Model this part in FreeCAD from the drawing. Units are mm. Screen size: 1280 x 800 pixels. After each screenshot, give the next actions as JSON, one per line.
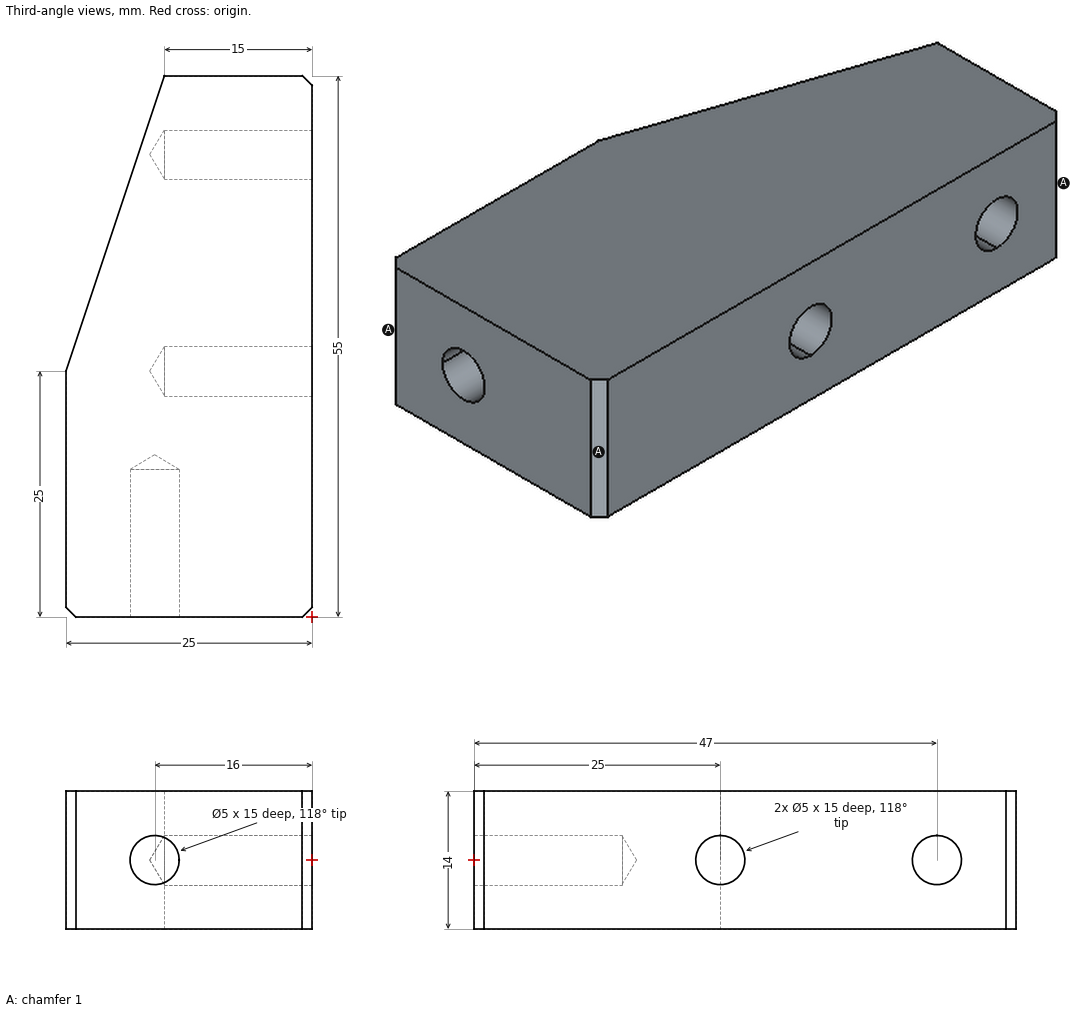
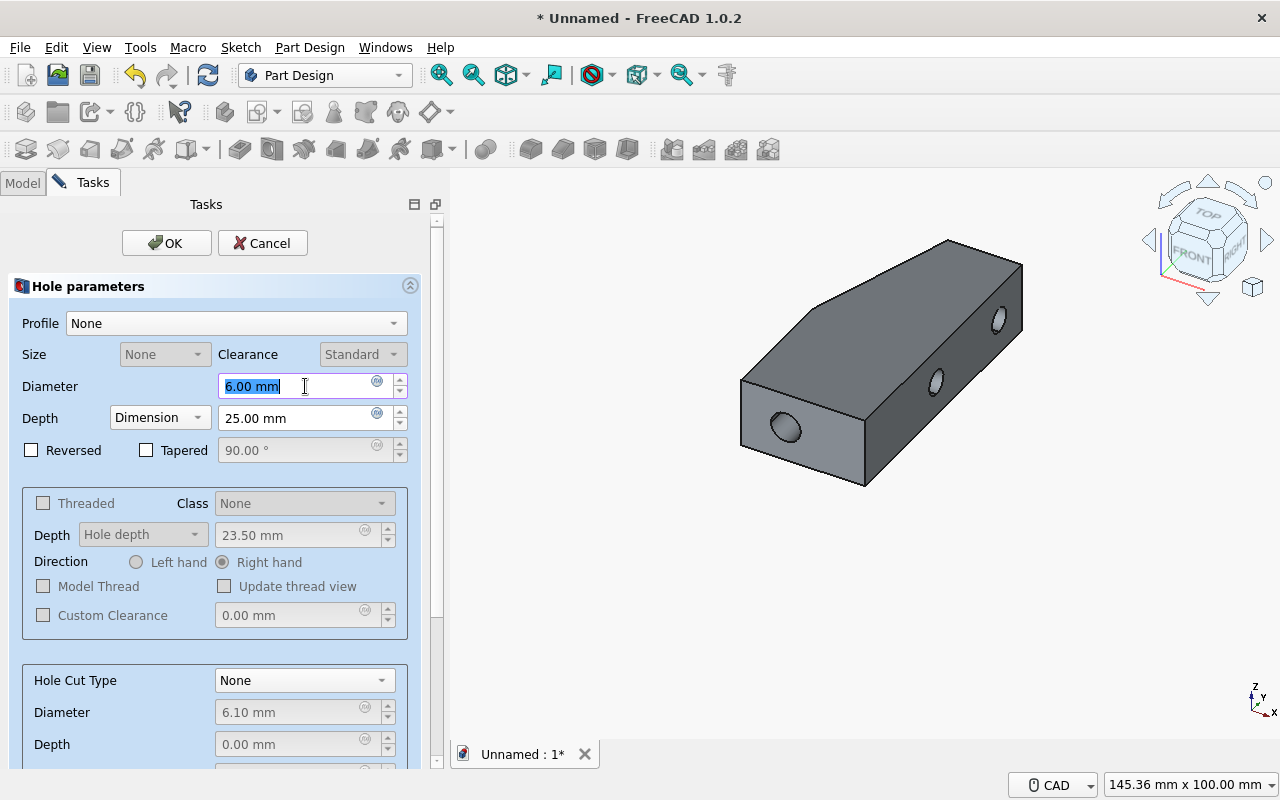
{"action": "type", "text": "5"}
{"action": "key", "text": "Tab"}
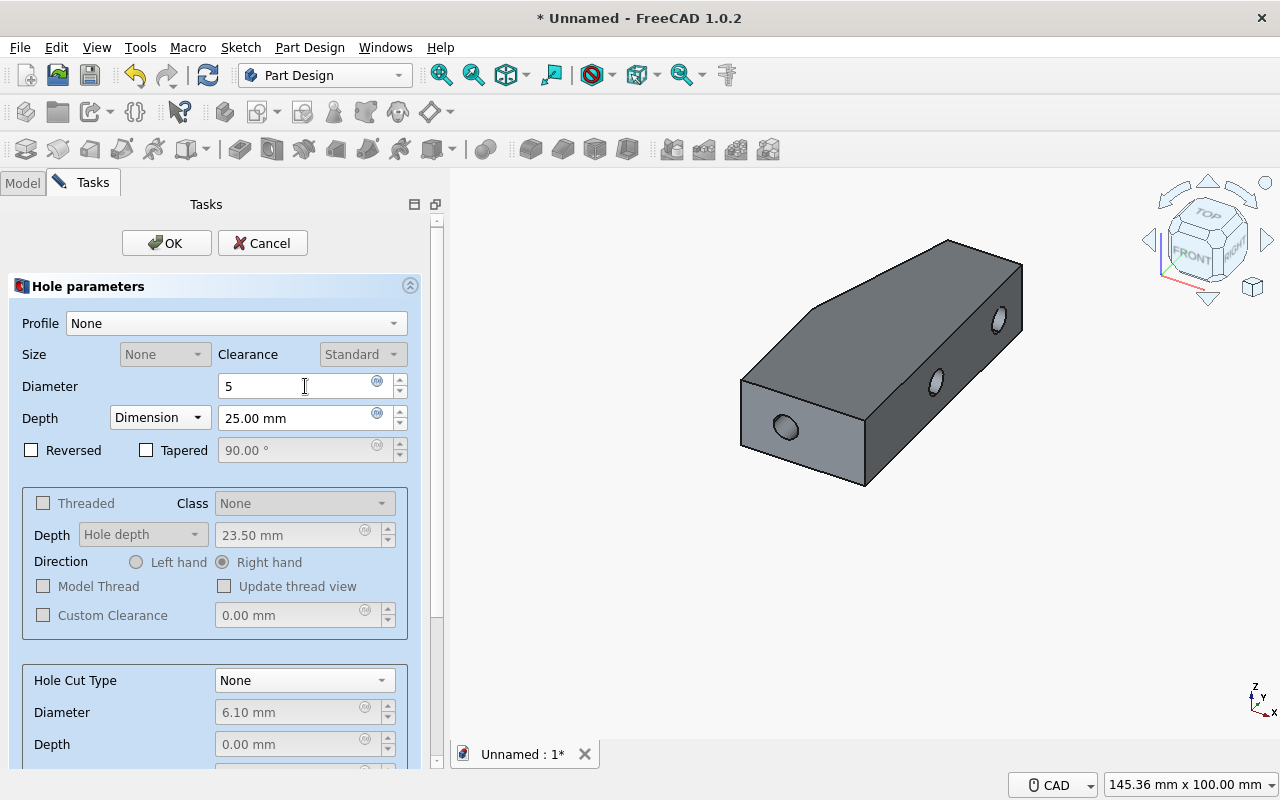
{"action": "triple_click", "coordinate": [305, 418]}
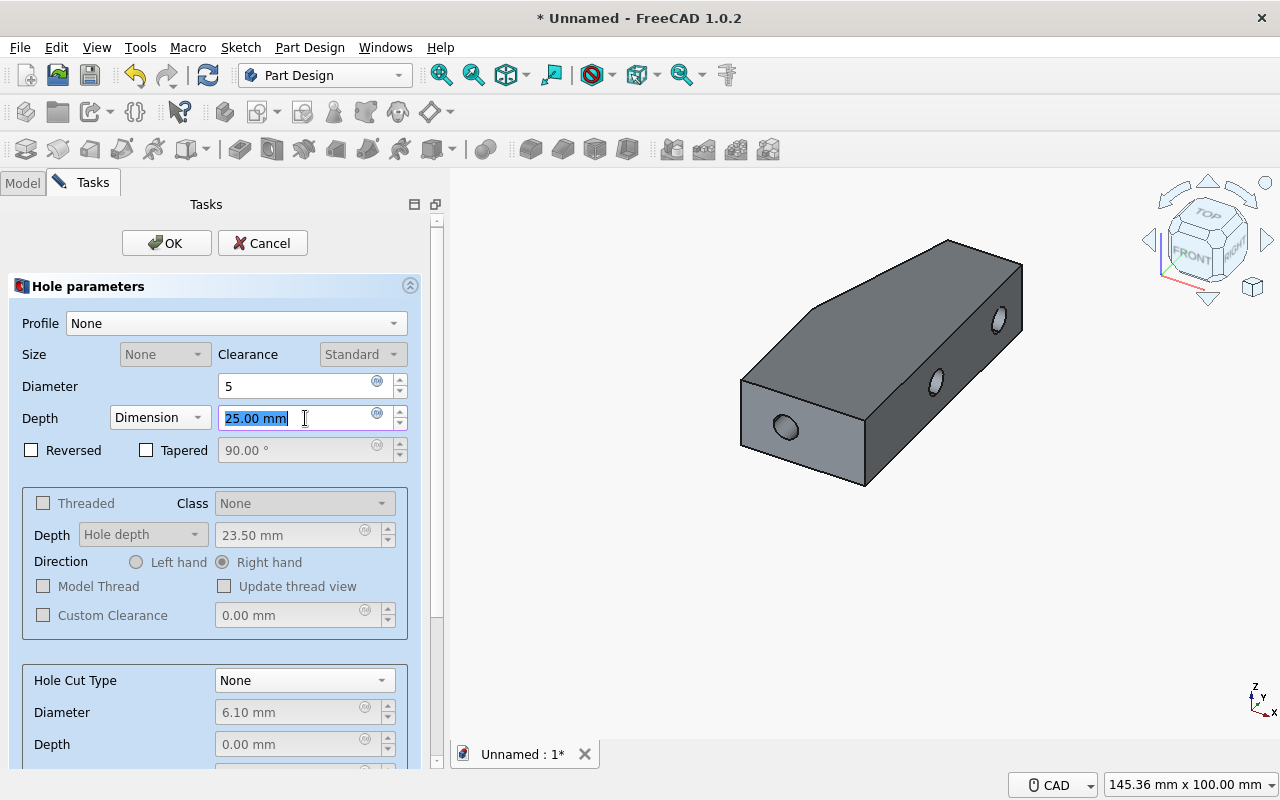
{"action": "type", "text": "15"}
{"action": "key", "text": "Tab"}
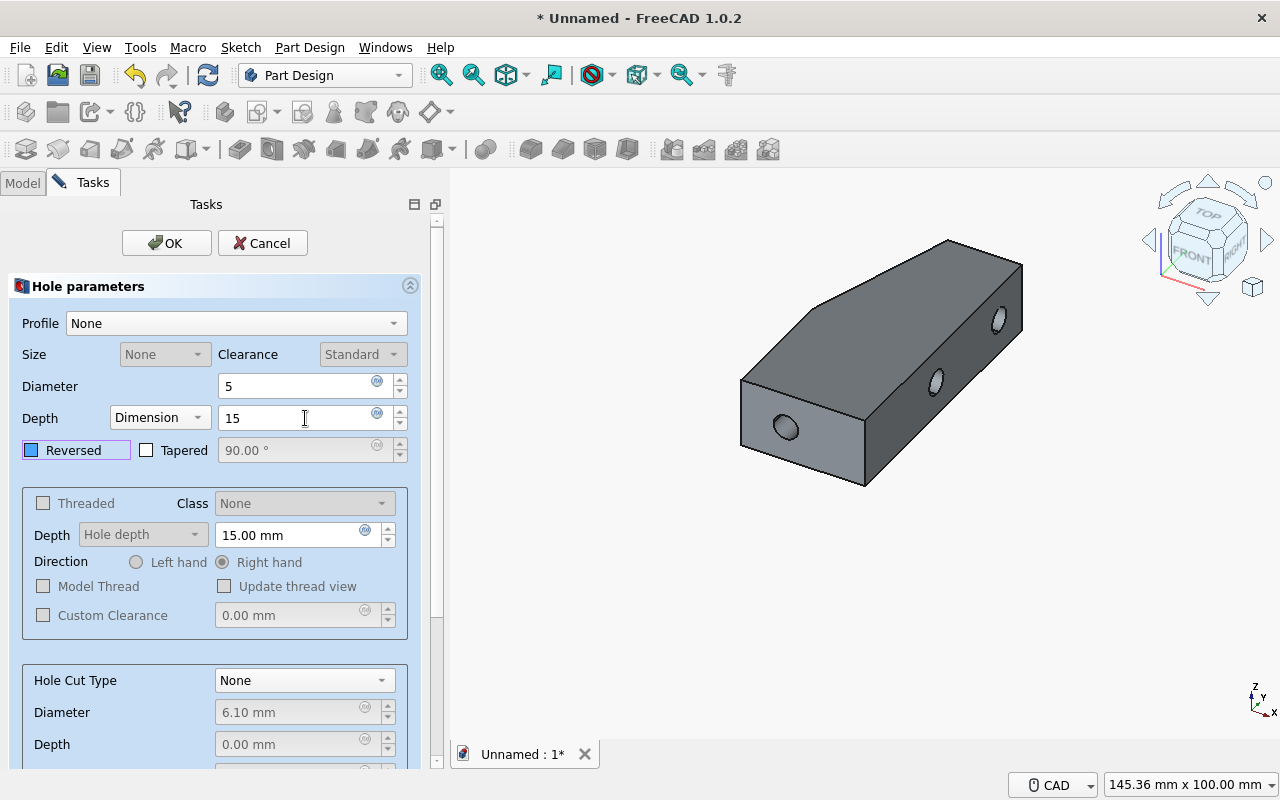
{"action": "left_click", "coordinate": [167, 243]}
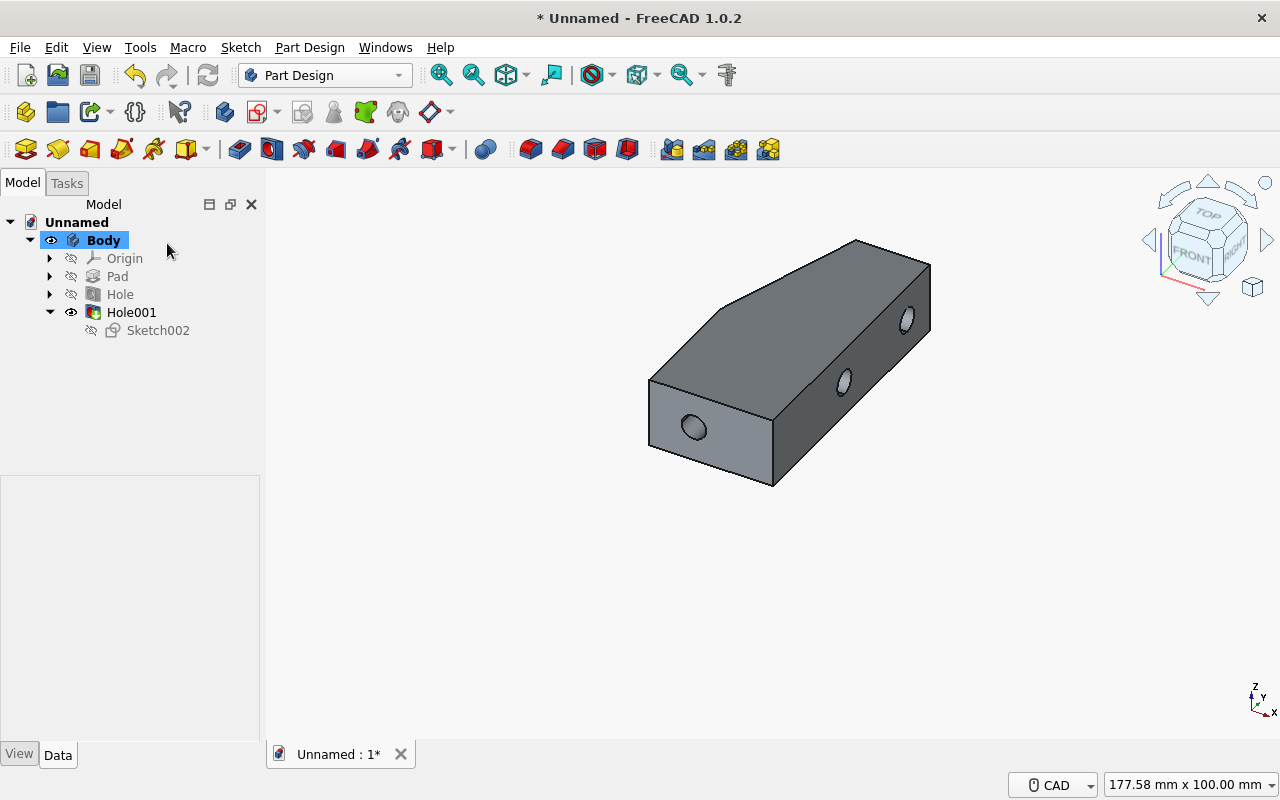
{"action": "left_click", "coordinate": [773, 452]}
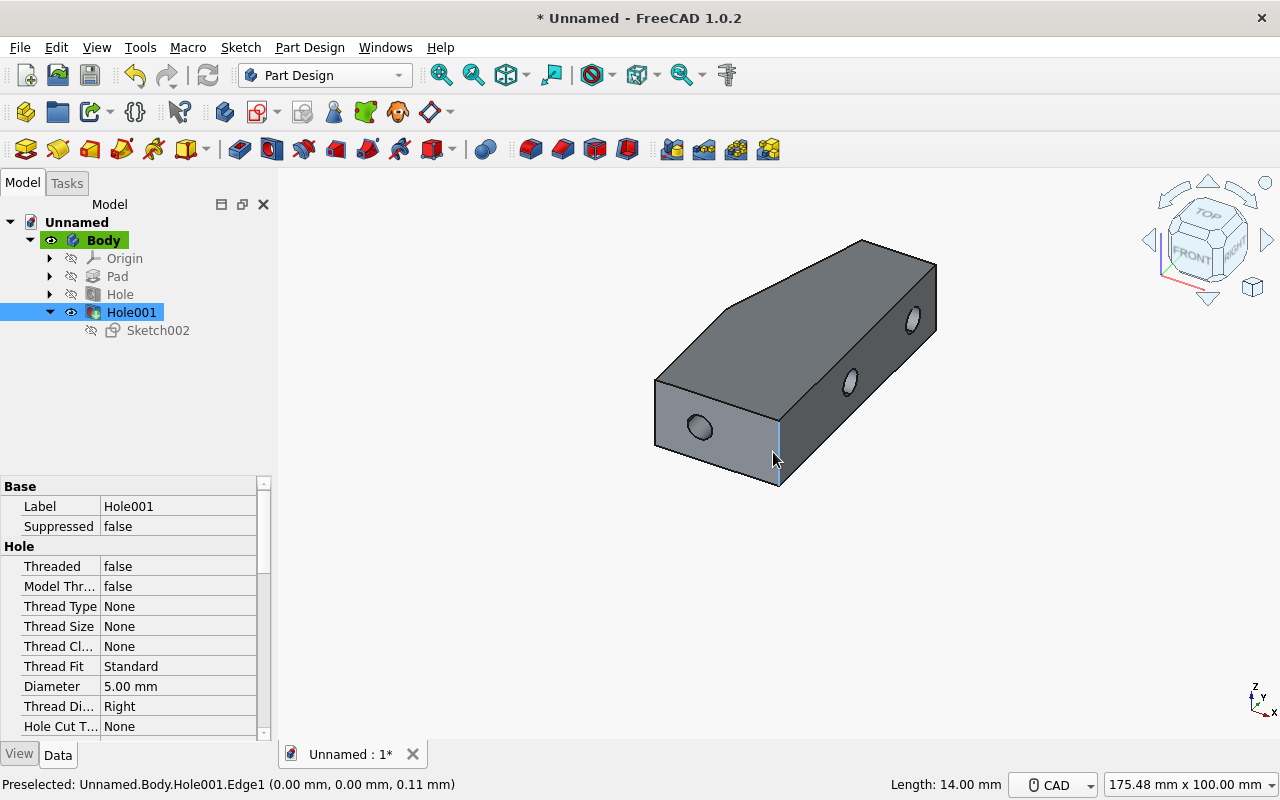
{"action": "key", "text": "0"}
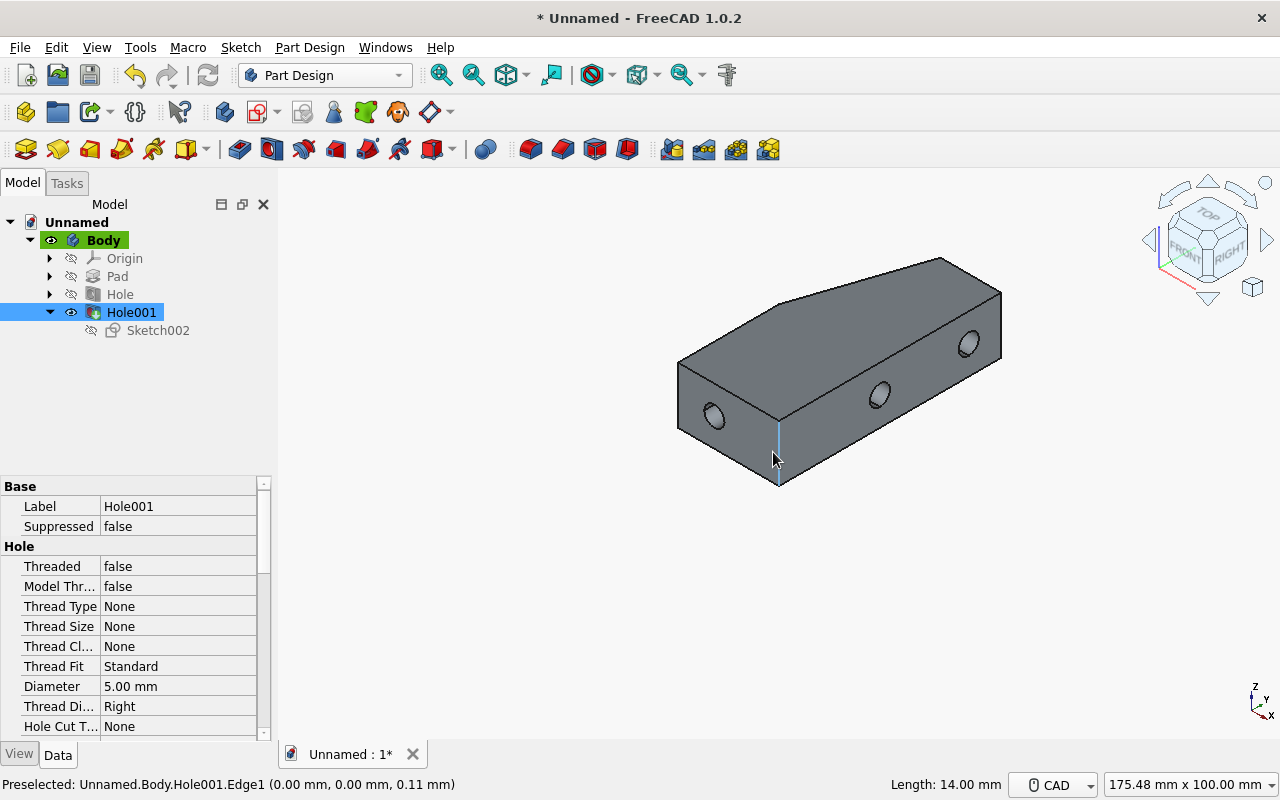
{"action": "key", "text": "v f"}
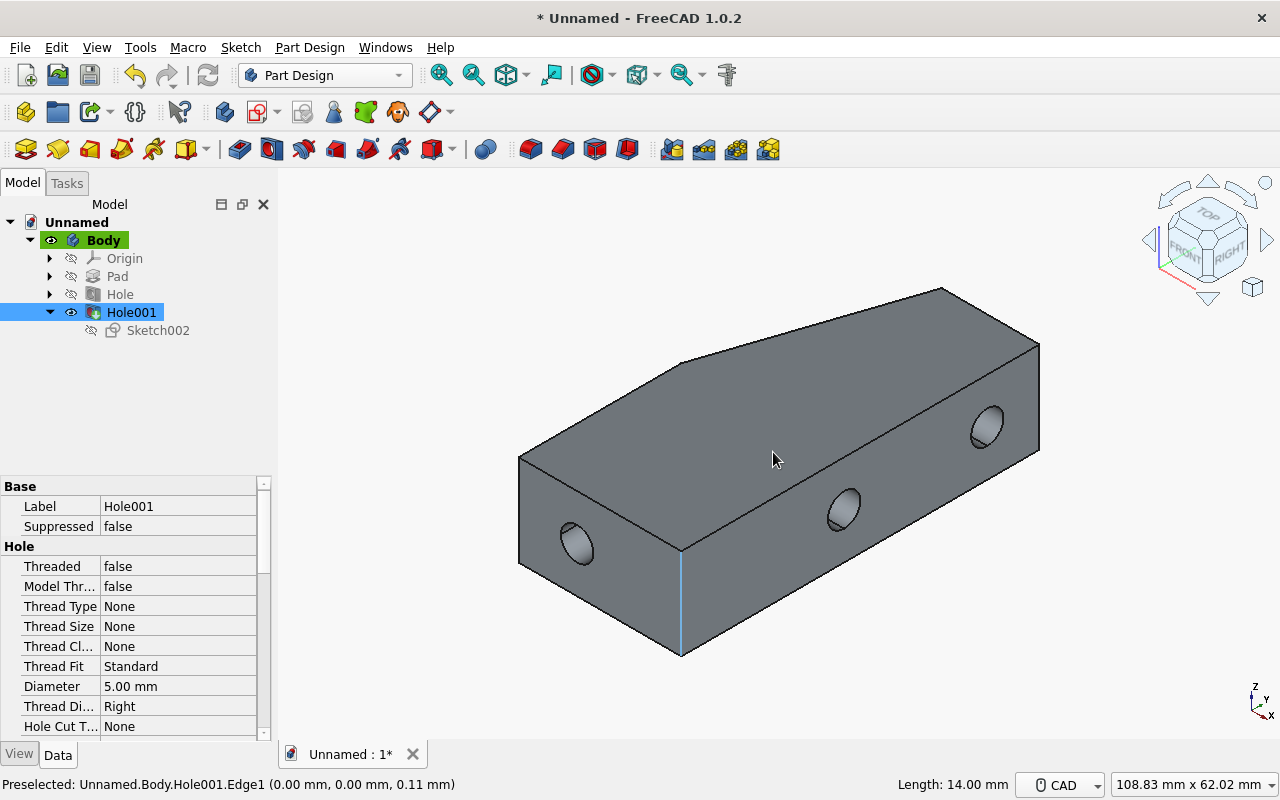
{"action": "key", "text": "2"}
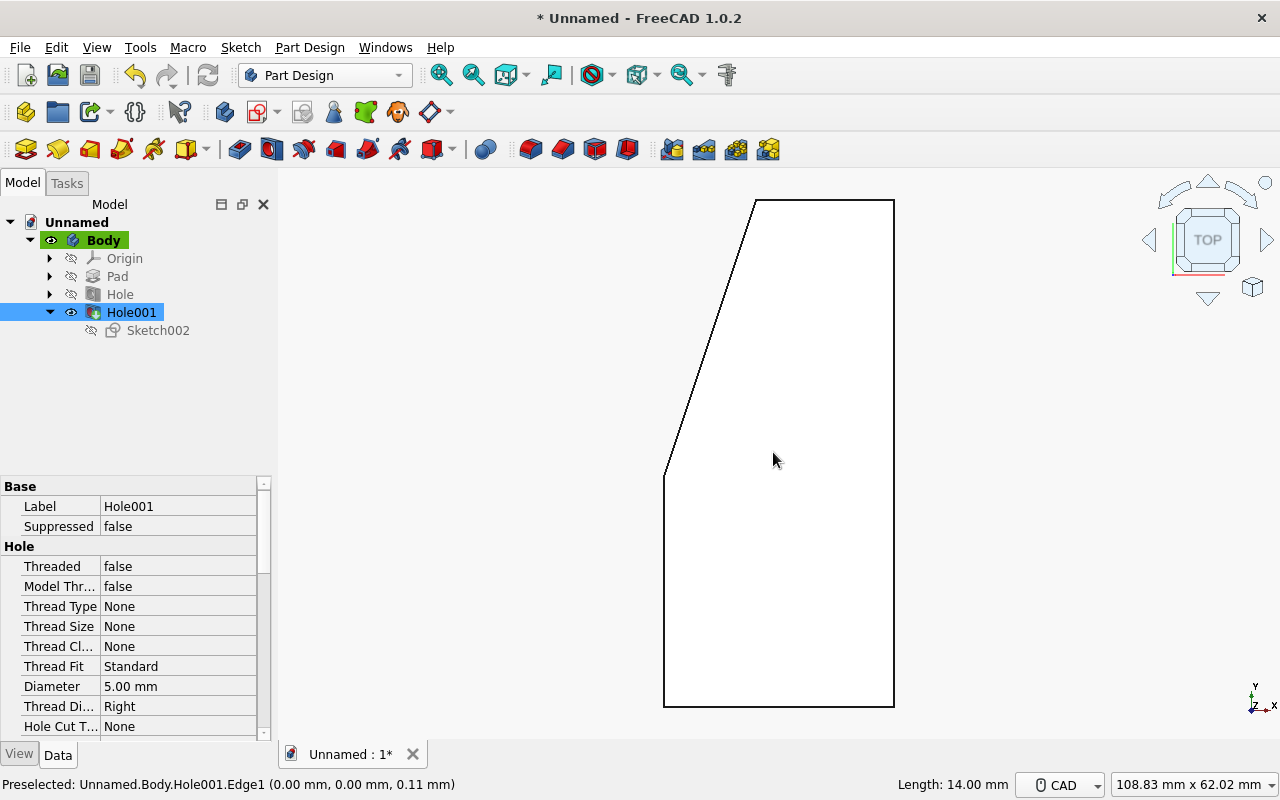
{"action": "key", "text": "1"}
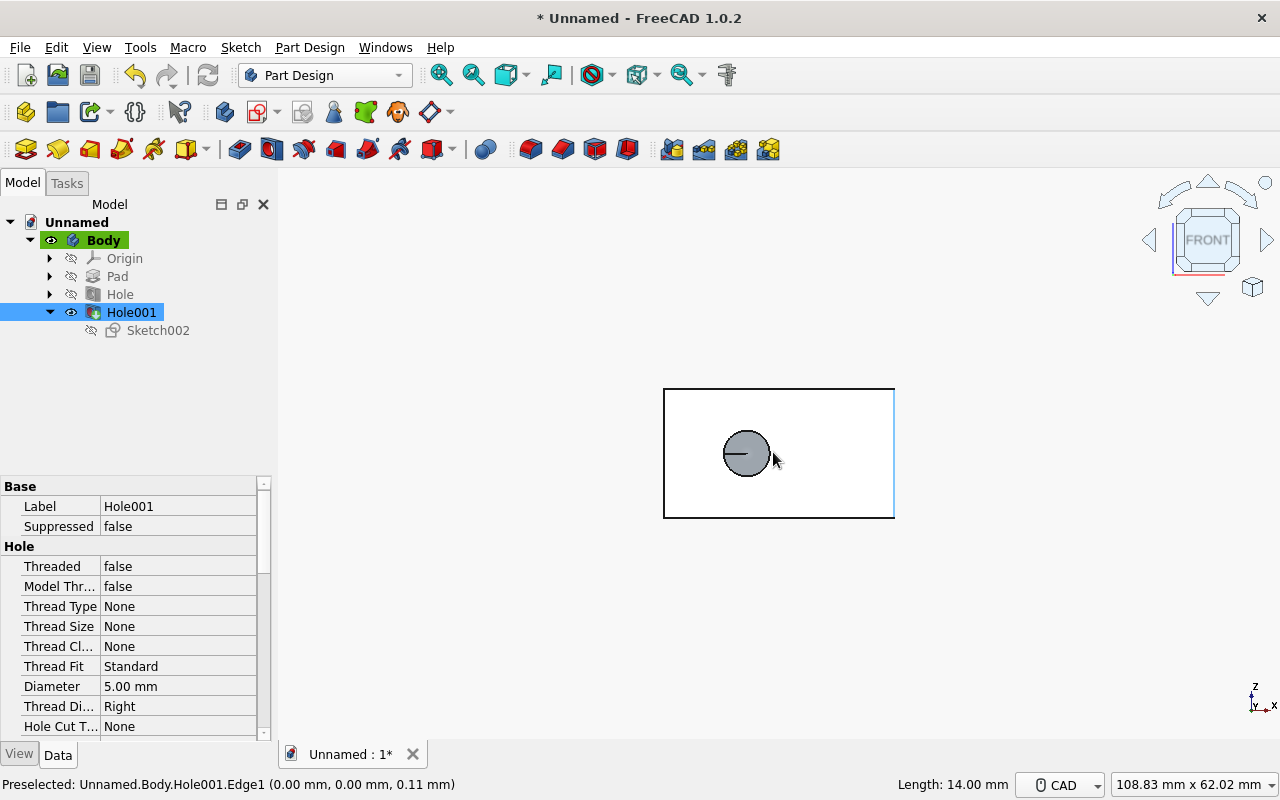
{"action": "key", "text": "v f"}